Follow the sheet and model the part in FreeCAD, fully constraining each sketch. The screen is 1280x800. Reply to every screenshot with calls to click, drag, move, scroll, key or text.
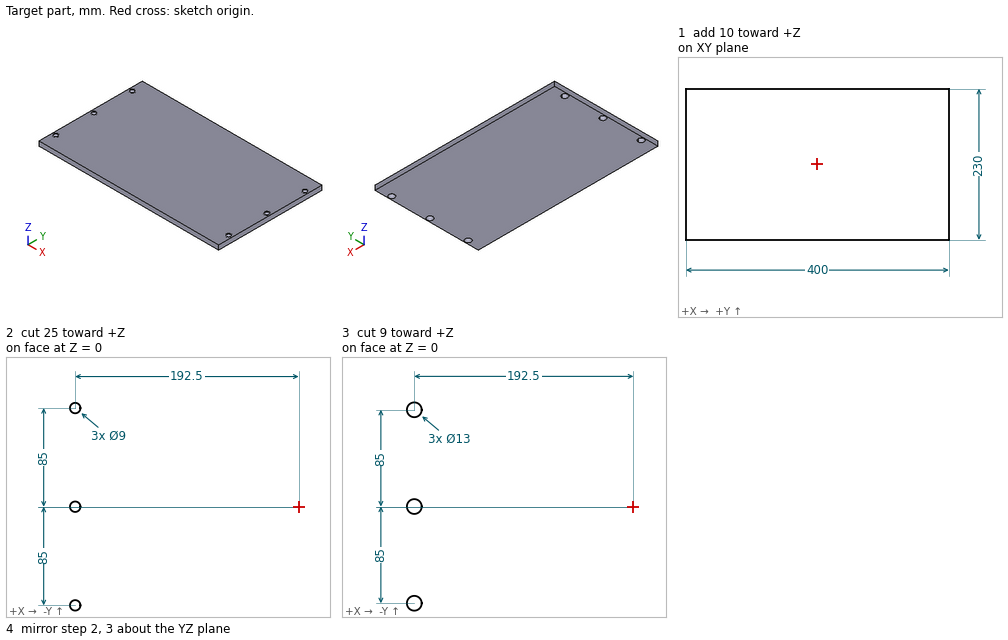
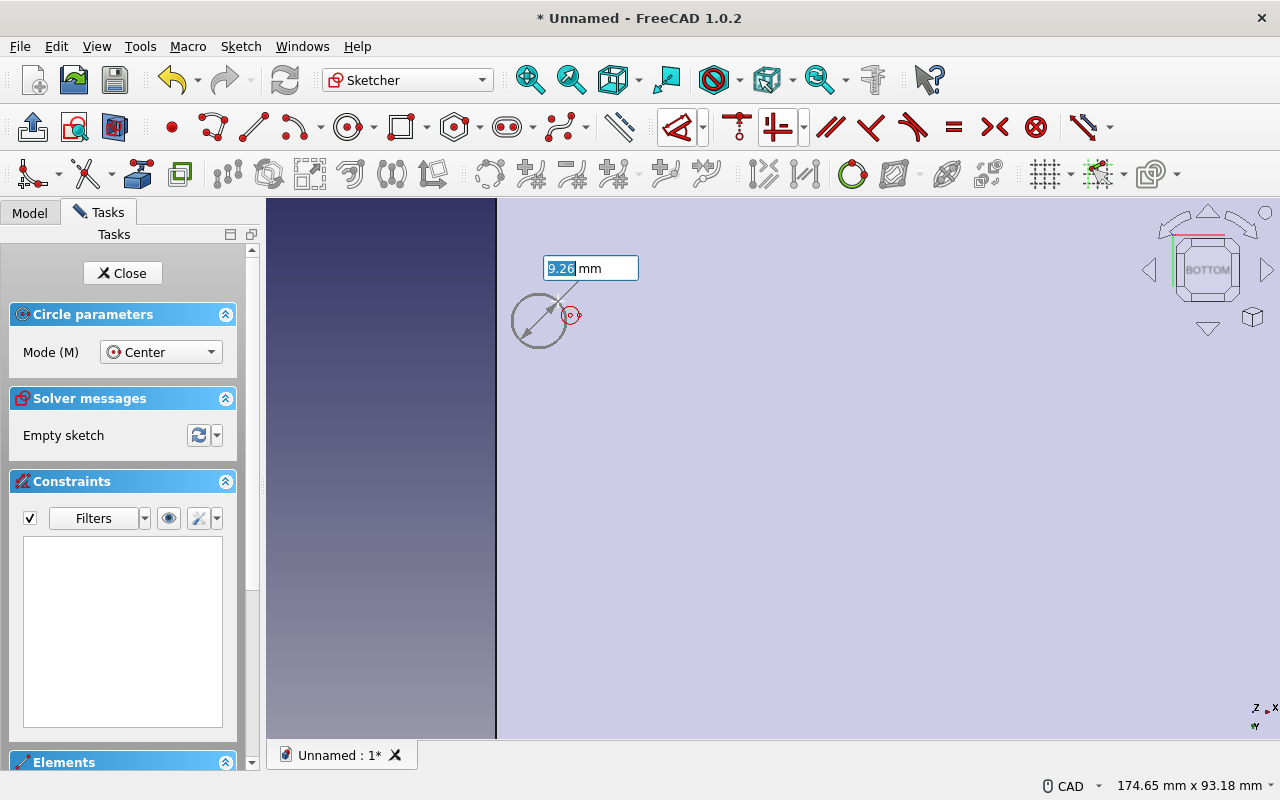
text(9)
key(Return)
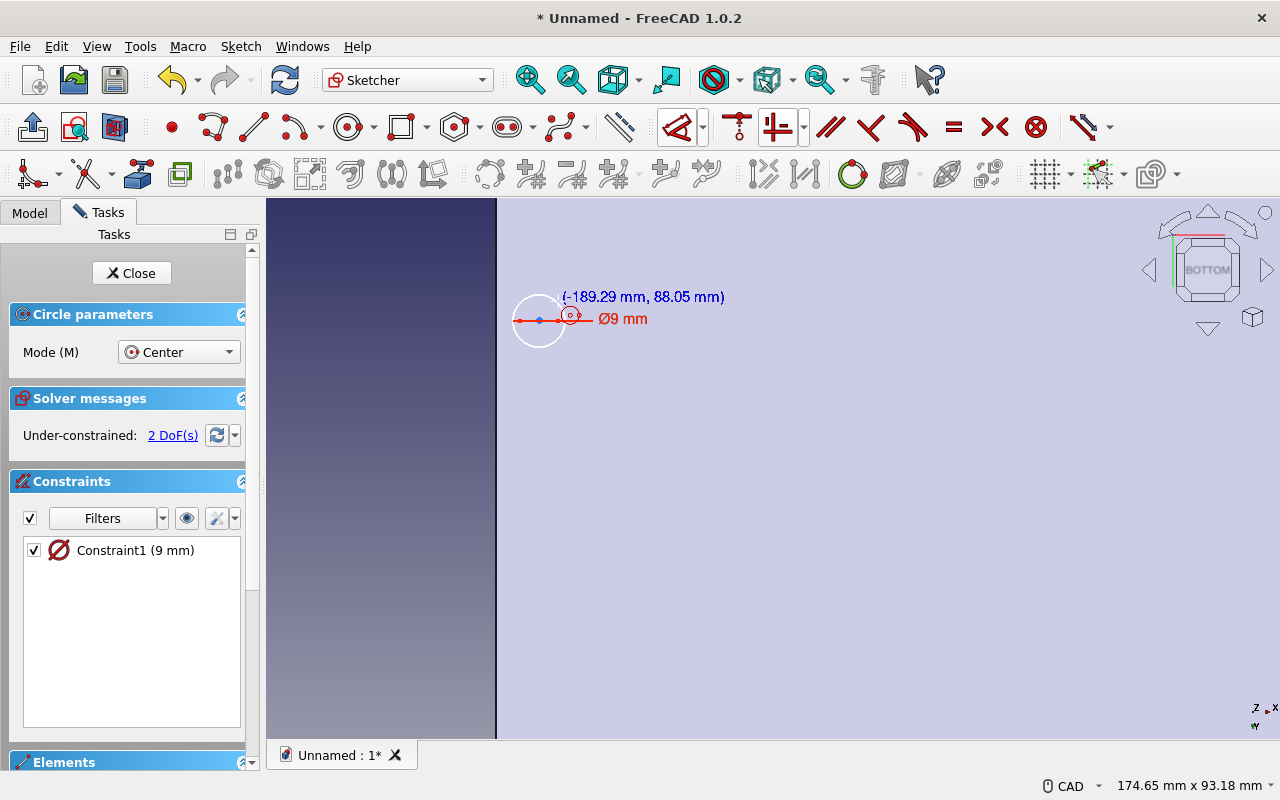
scroll(540, 320, down, 6)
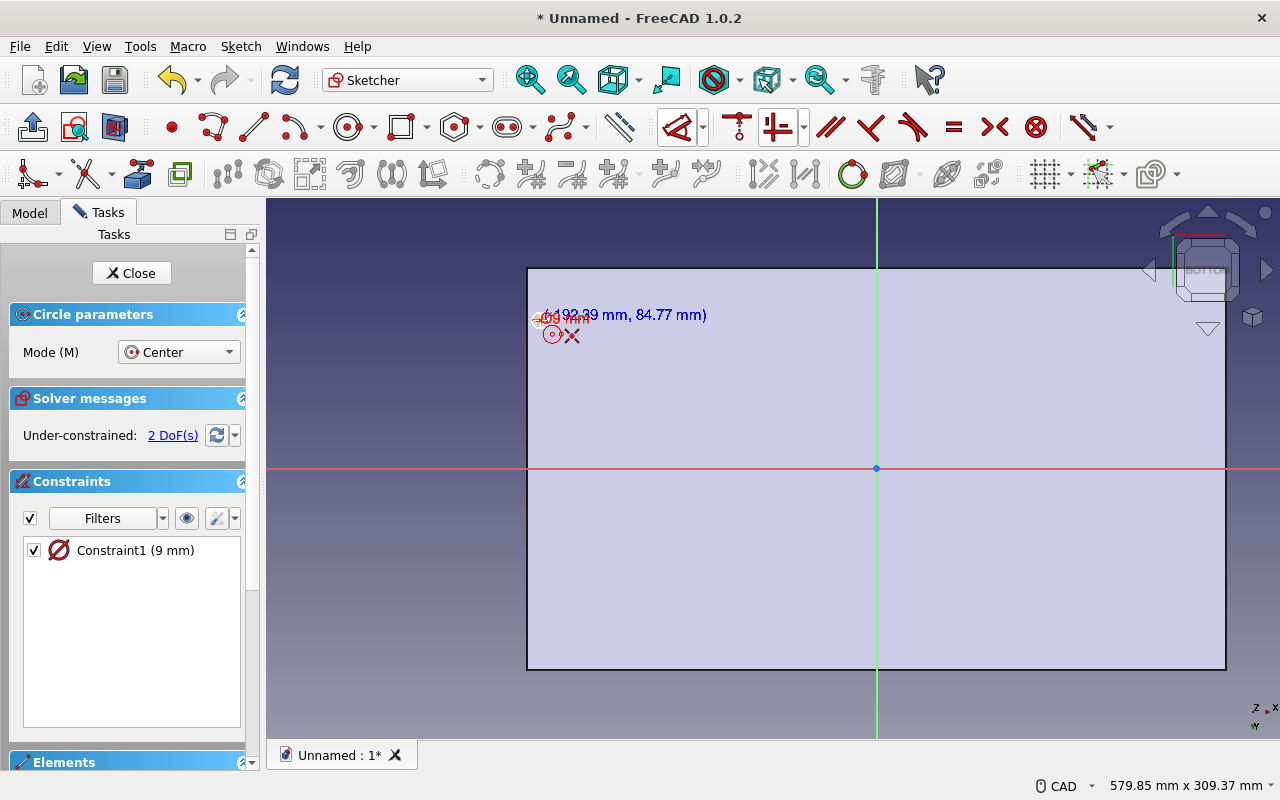
scroll(540, 469, up, 6)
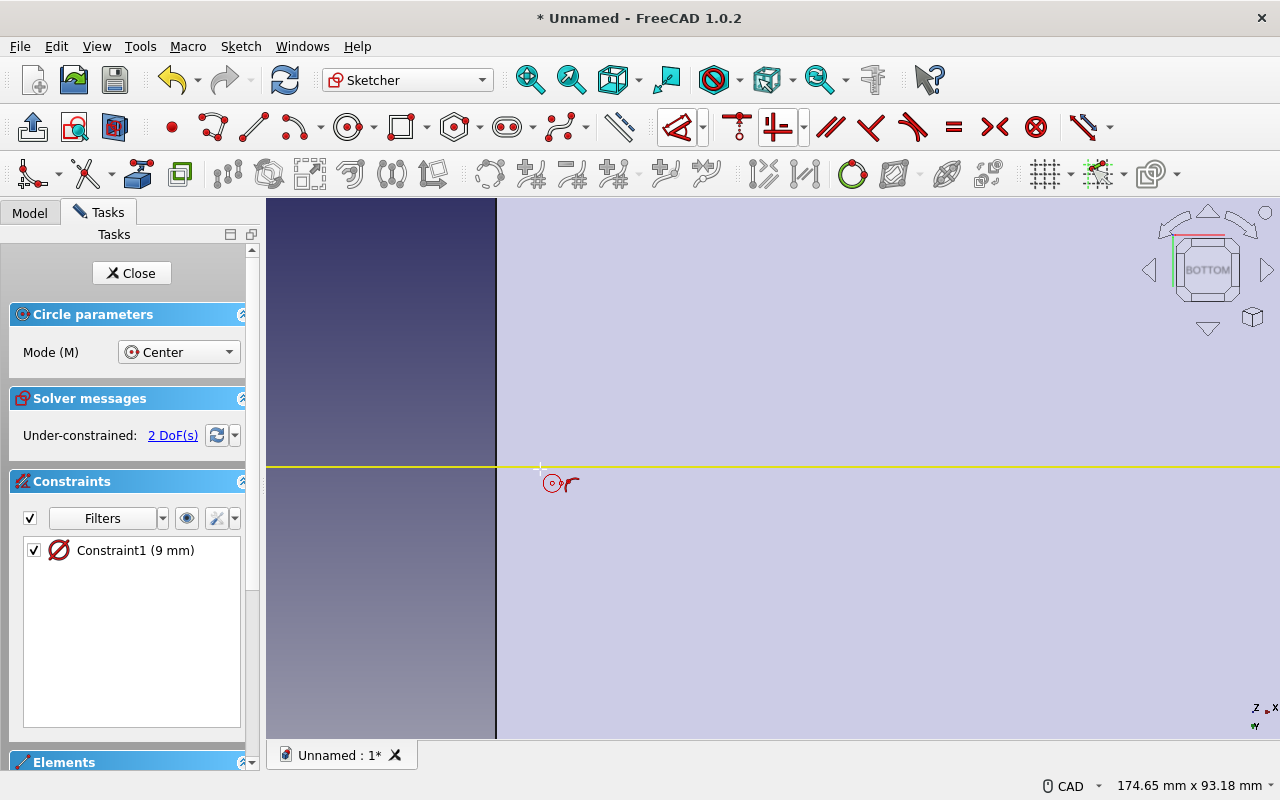
click(539, 467)
move(558, 448)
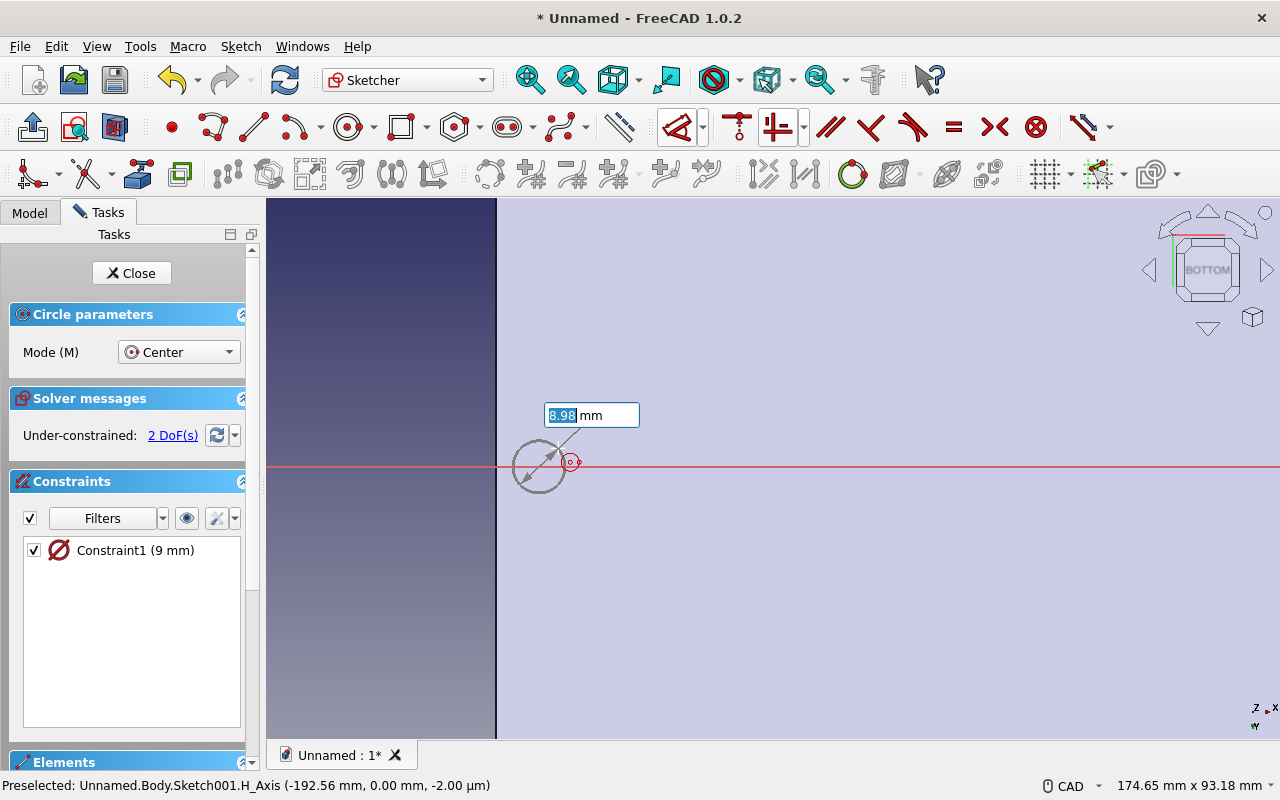
text(9)
key(Return)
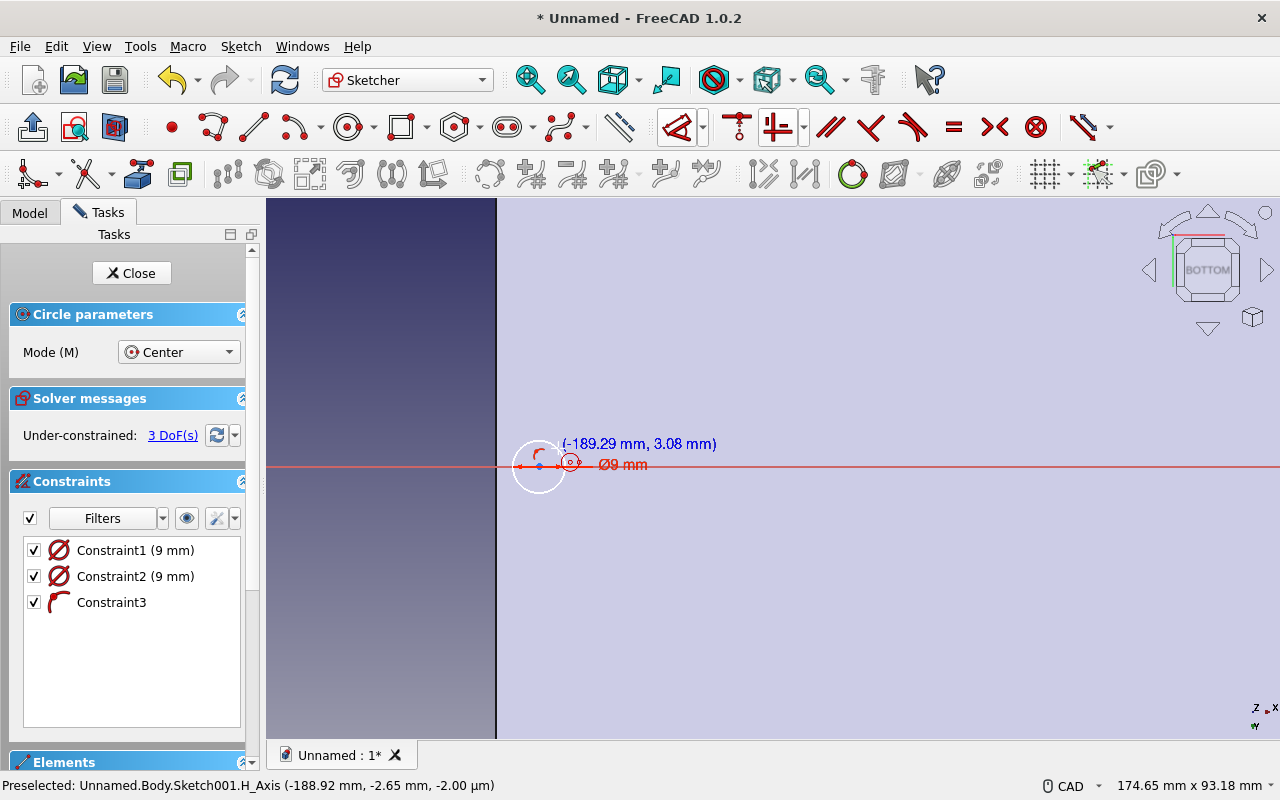
scroll(540, 469, down, 6)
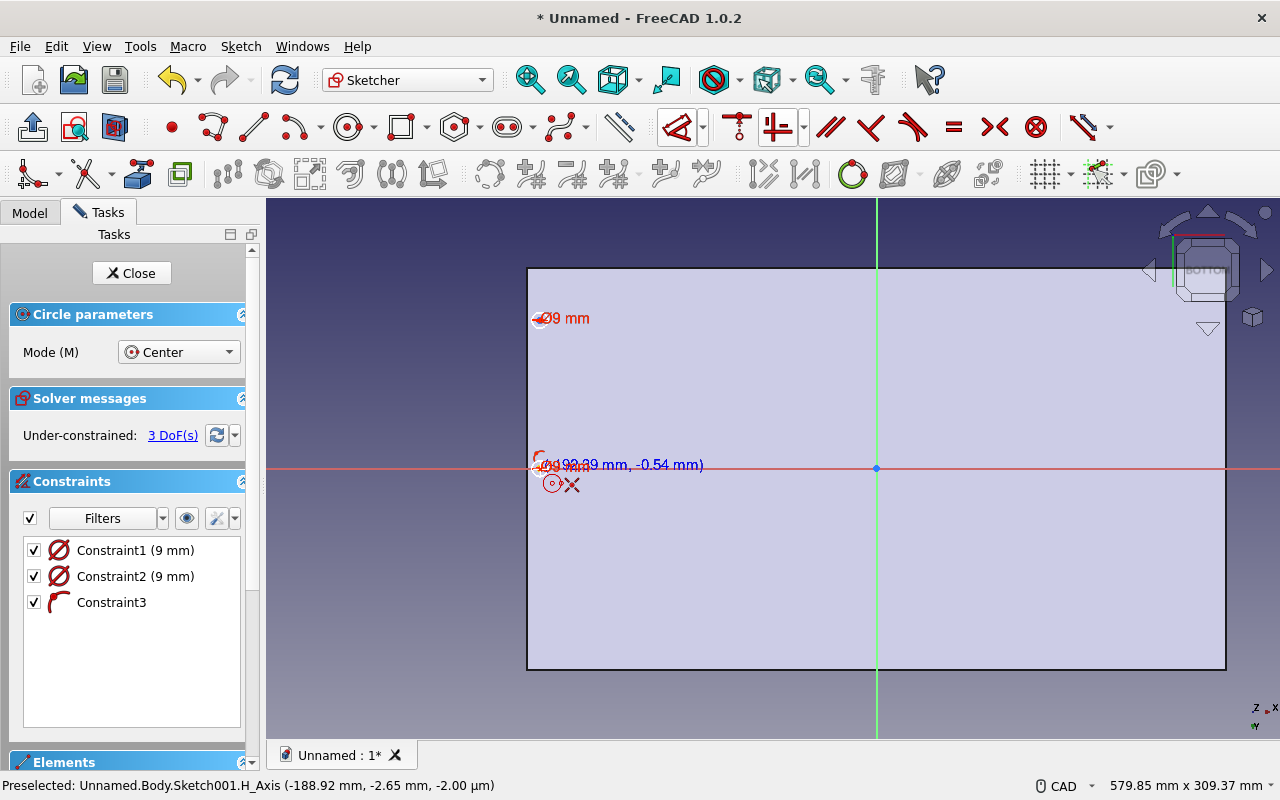
scroll(540, 617, up, 6)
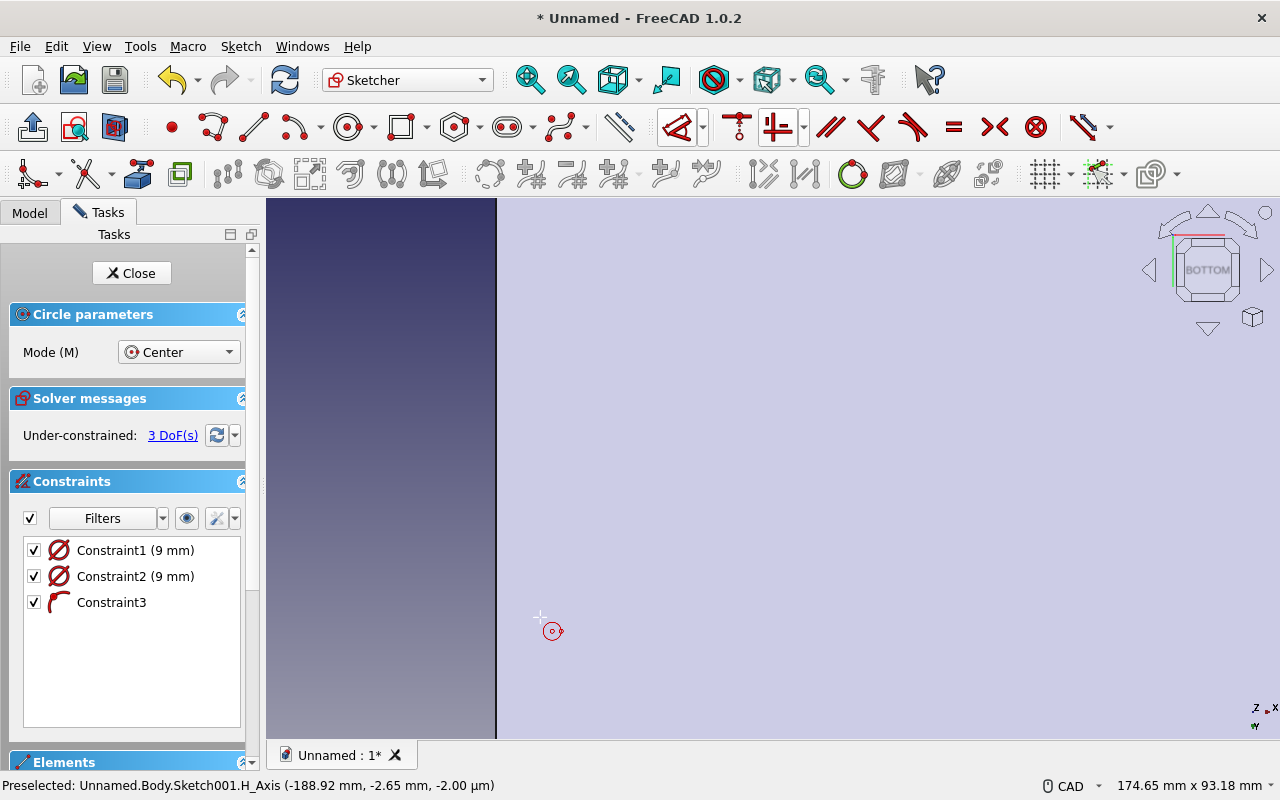
click(539, 616)
move(558, 598)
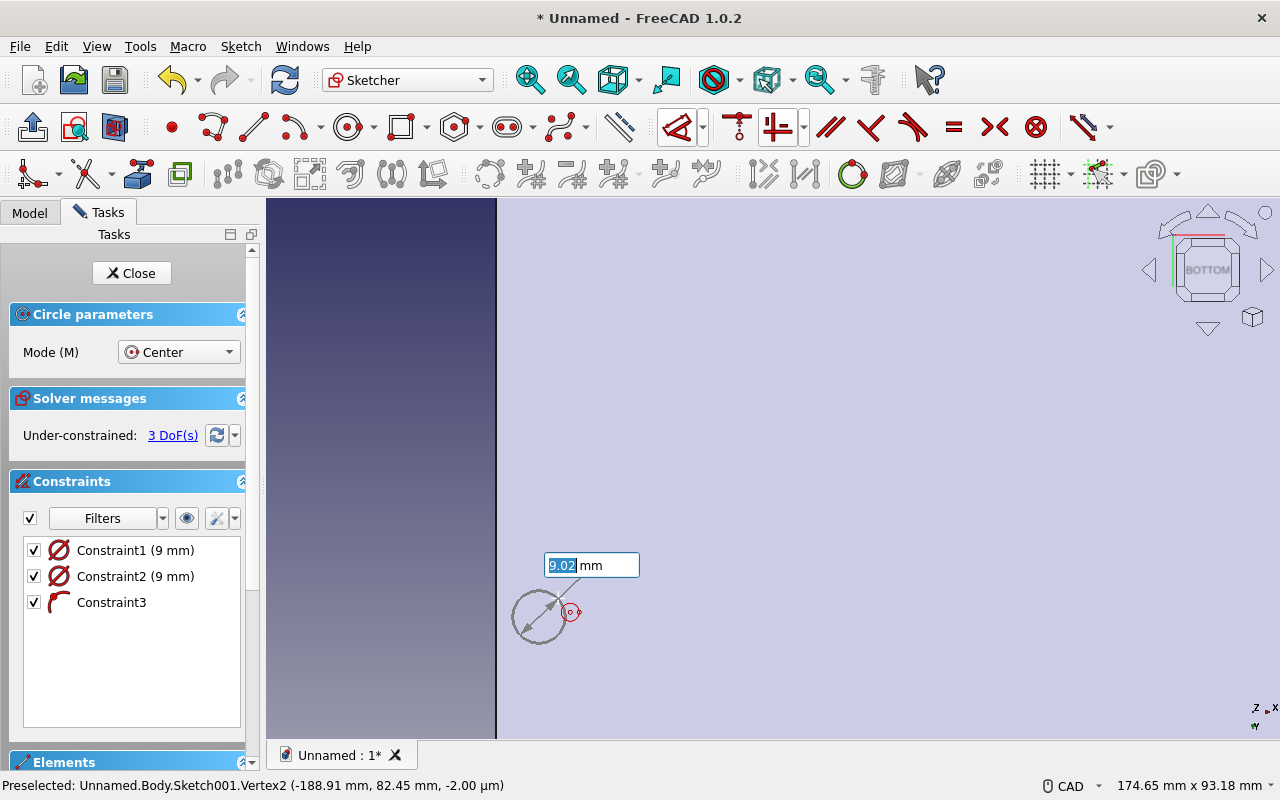
text(9)
key(Return)
key(Escape)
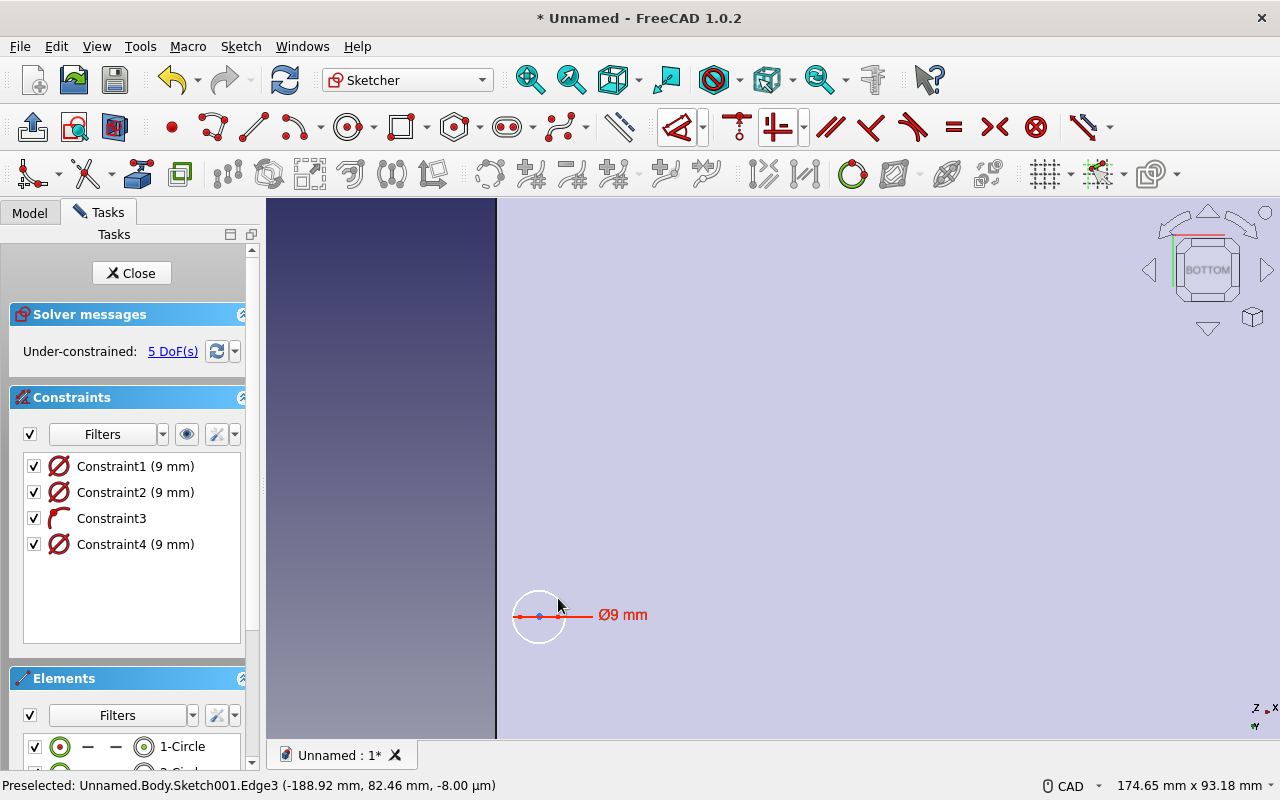
scroll(540, 617, down, 6)